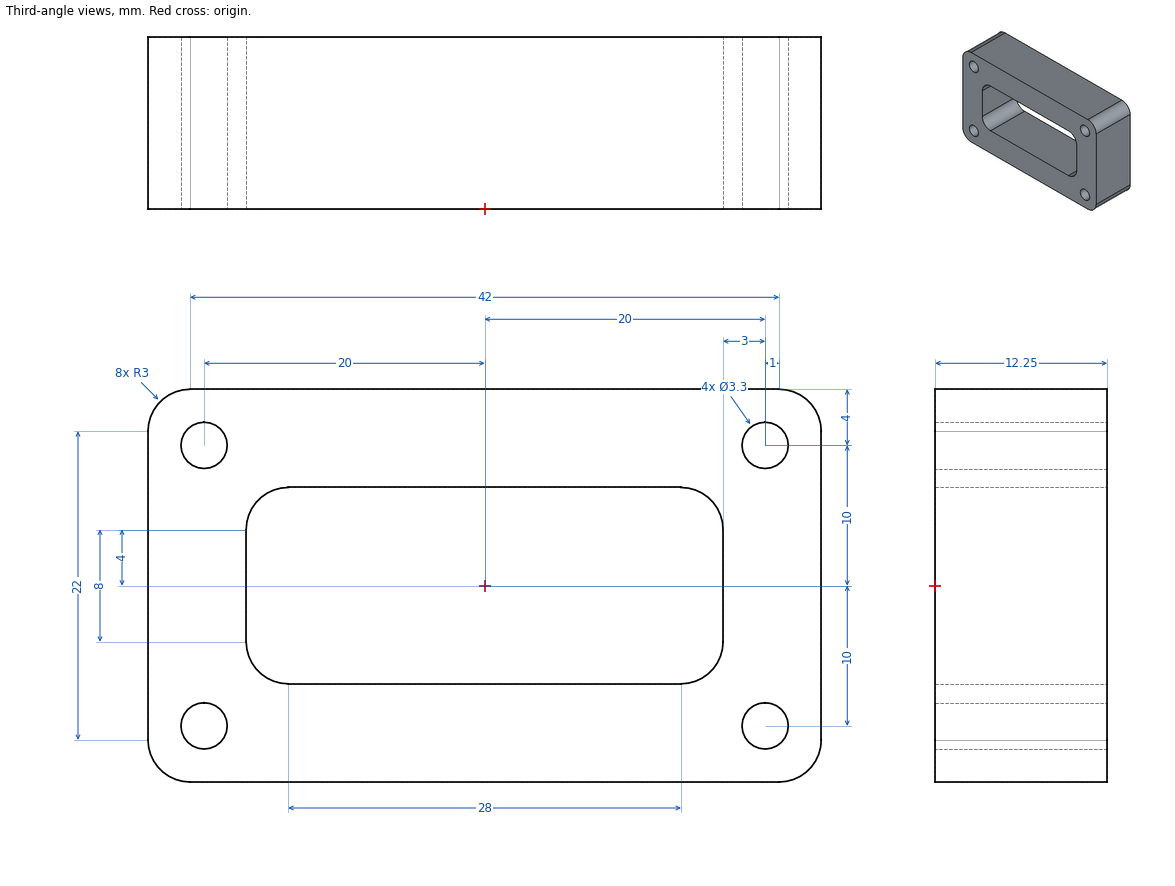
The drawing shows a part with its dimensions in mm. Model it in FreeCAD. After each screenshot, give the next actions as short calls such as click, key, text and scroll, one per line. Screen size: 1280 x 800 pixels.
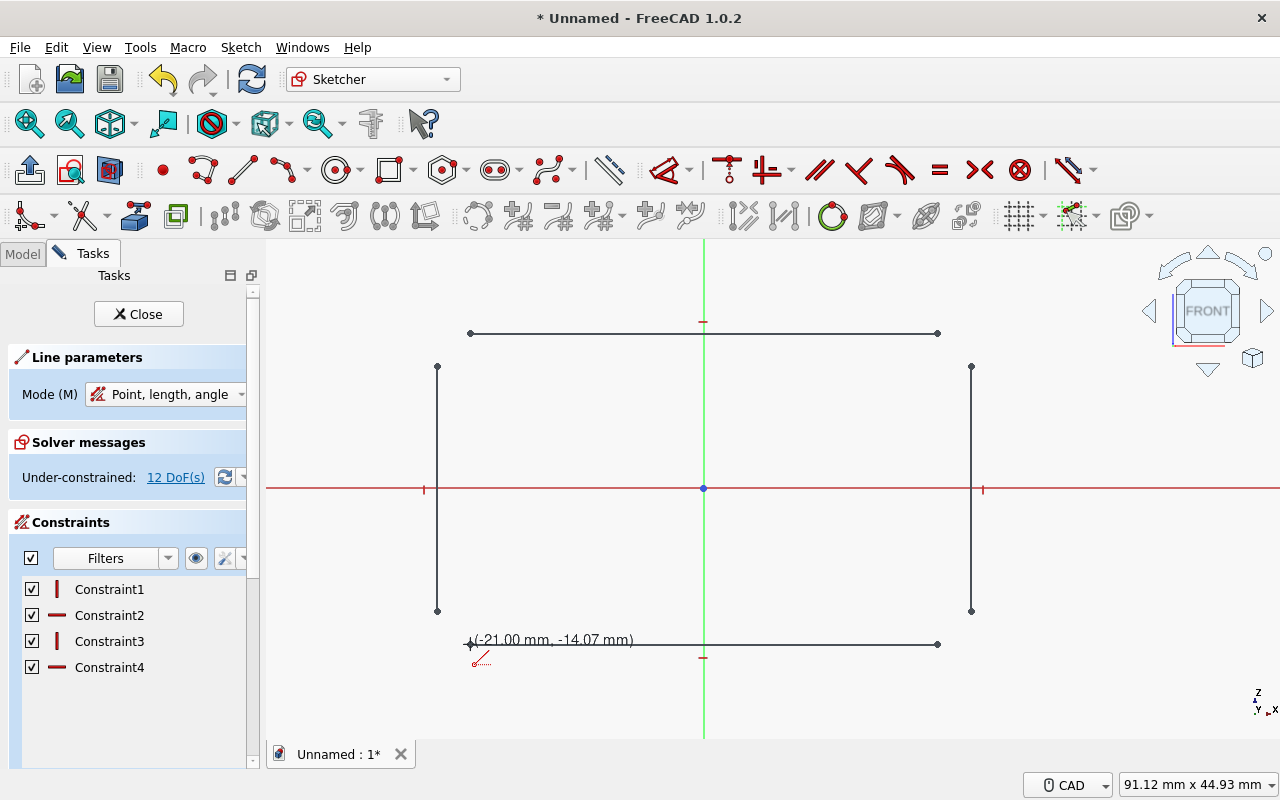
click(284, 170)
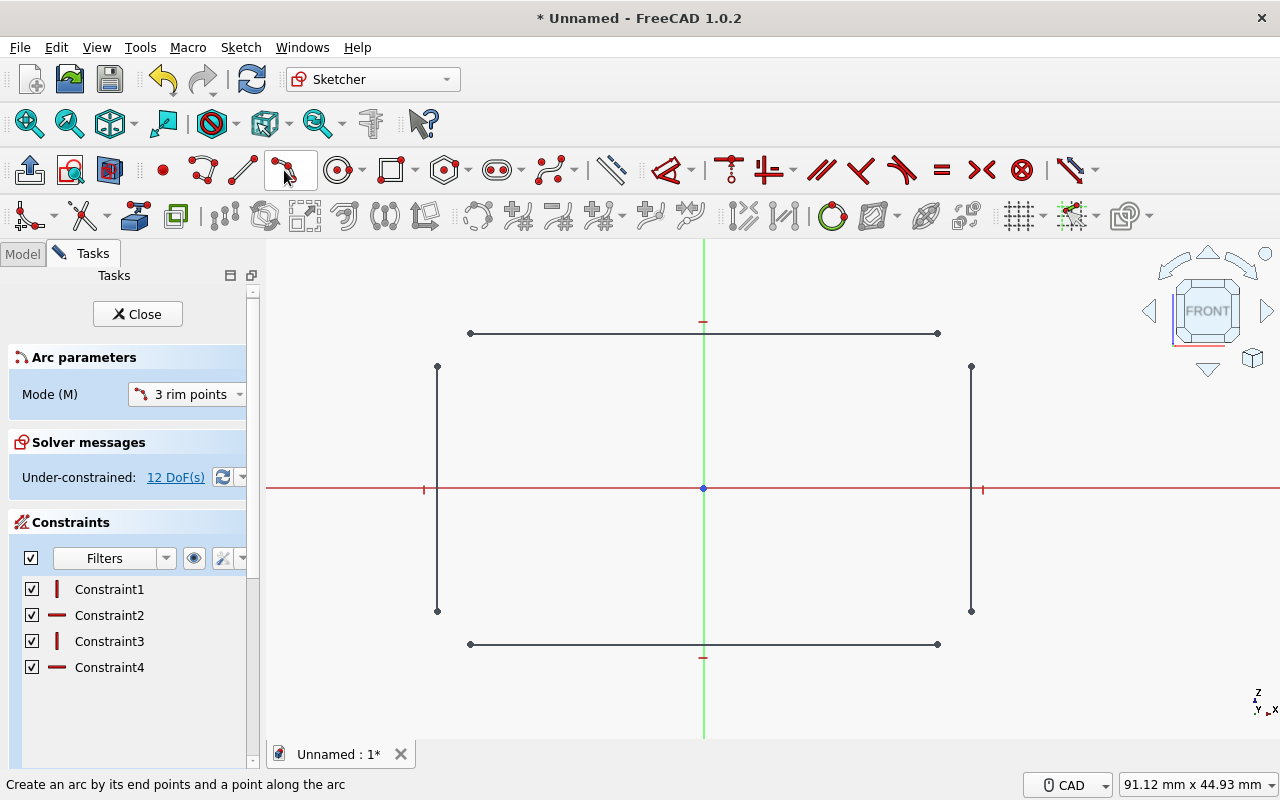
click(437, 367)
click(470, 334)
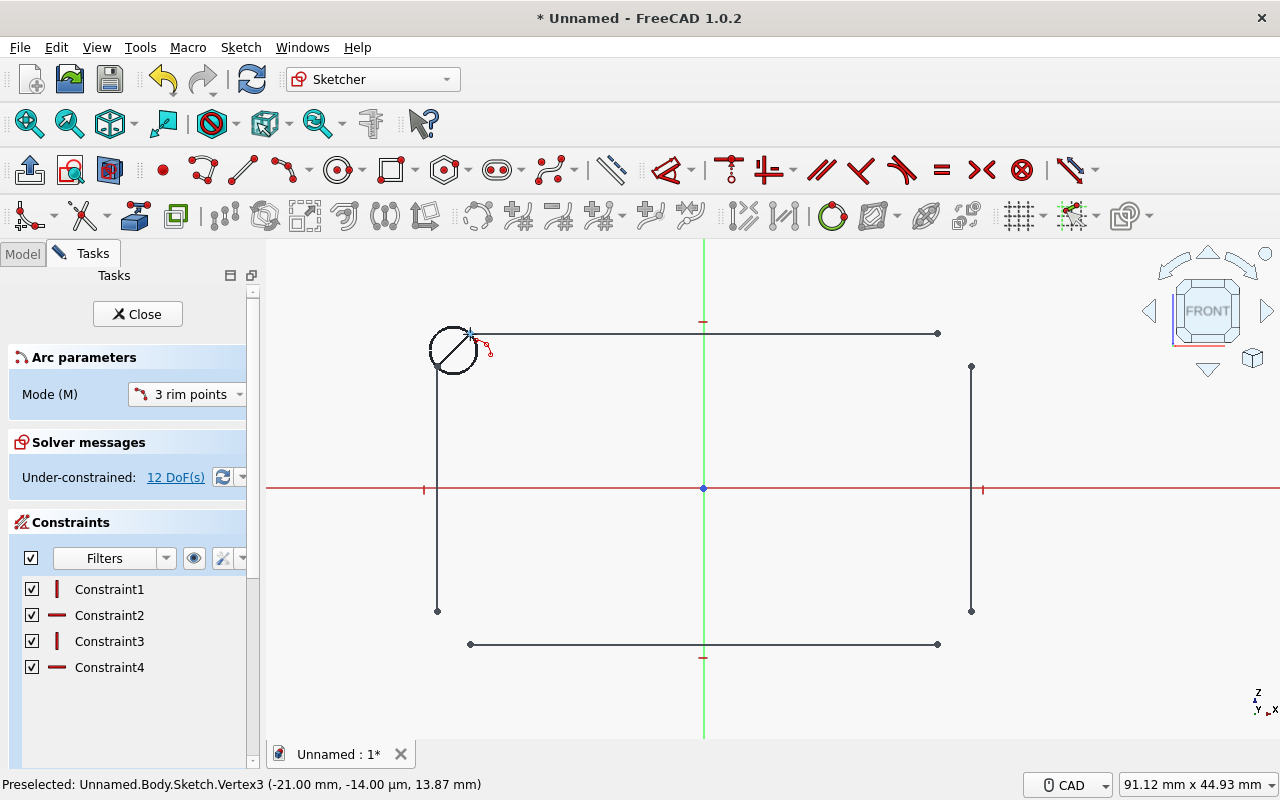
scroll(446, 342, up, 3)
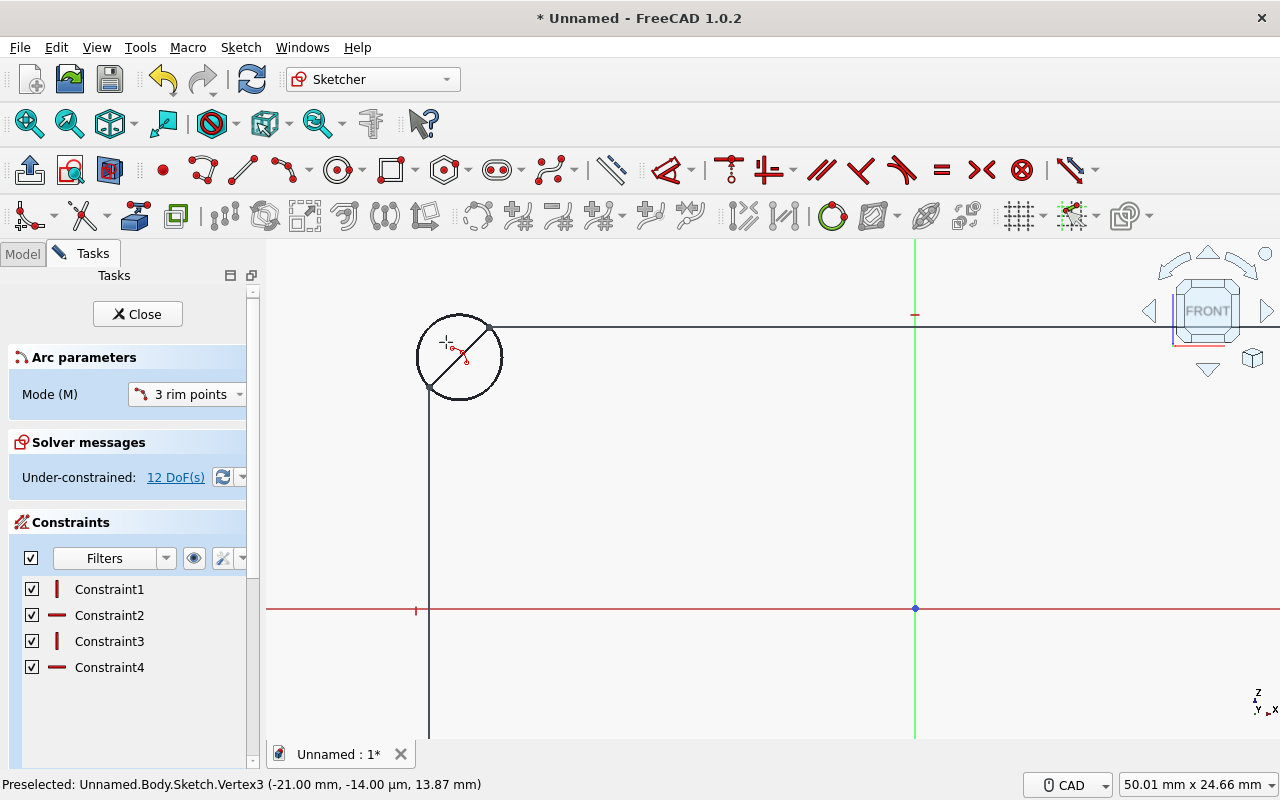
click(447, 343)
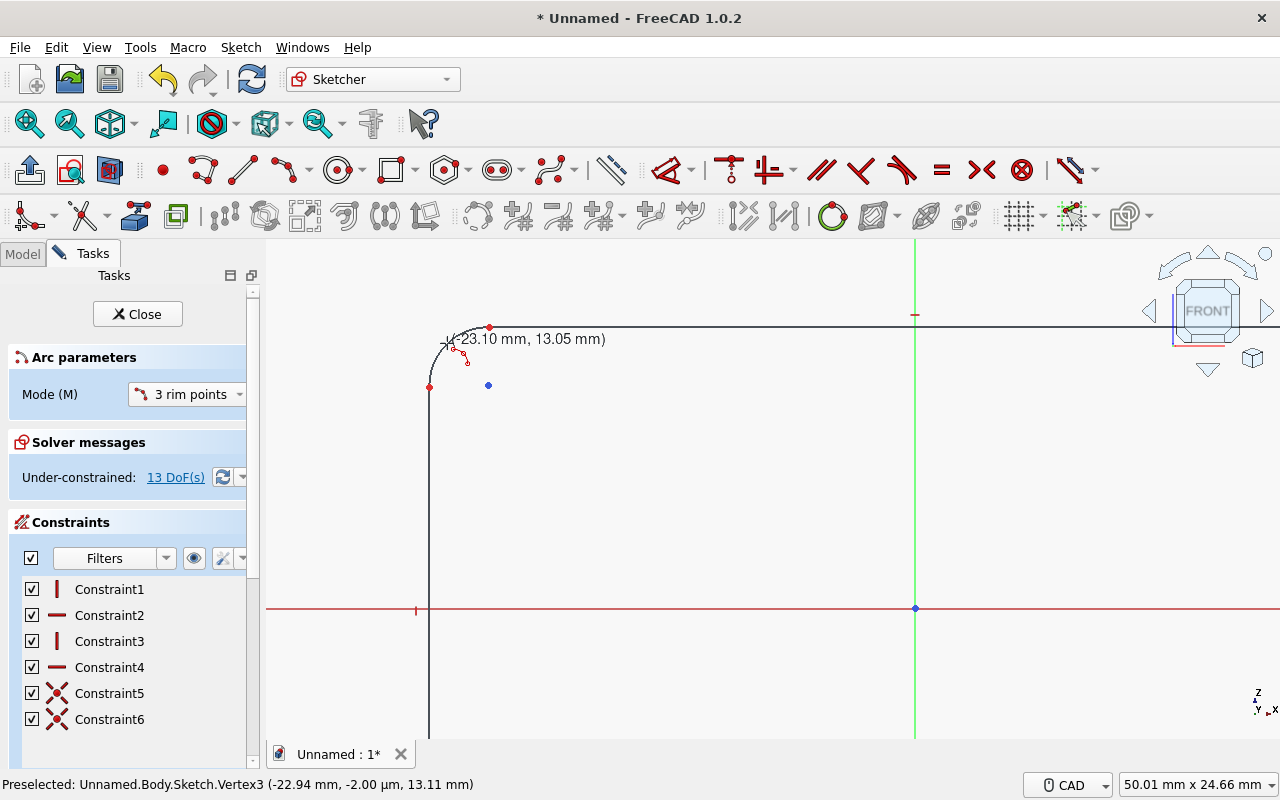
scroll(448, 344, down, 3)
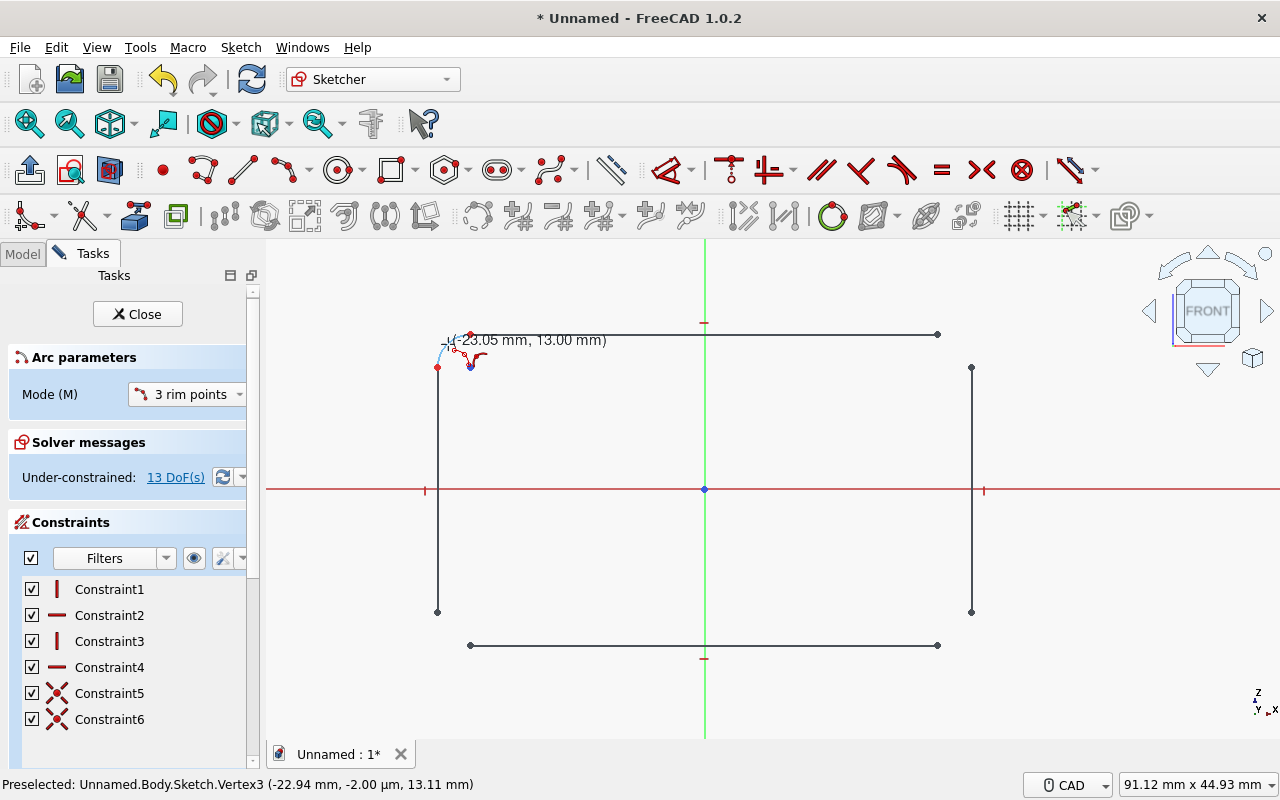
click(938, 335)
click(972, 368)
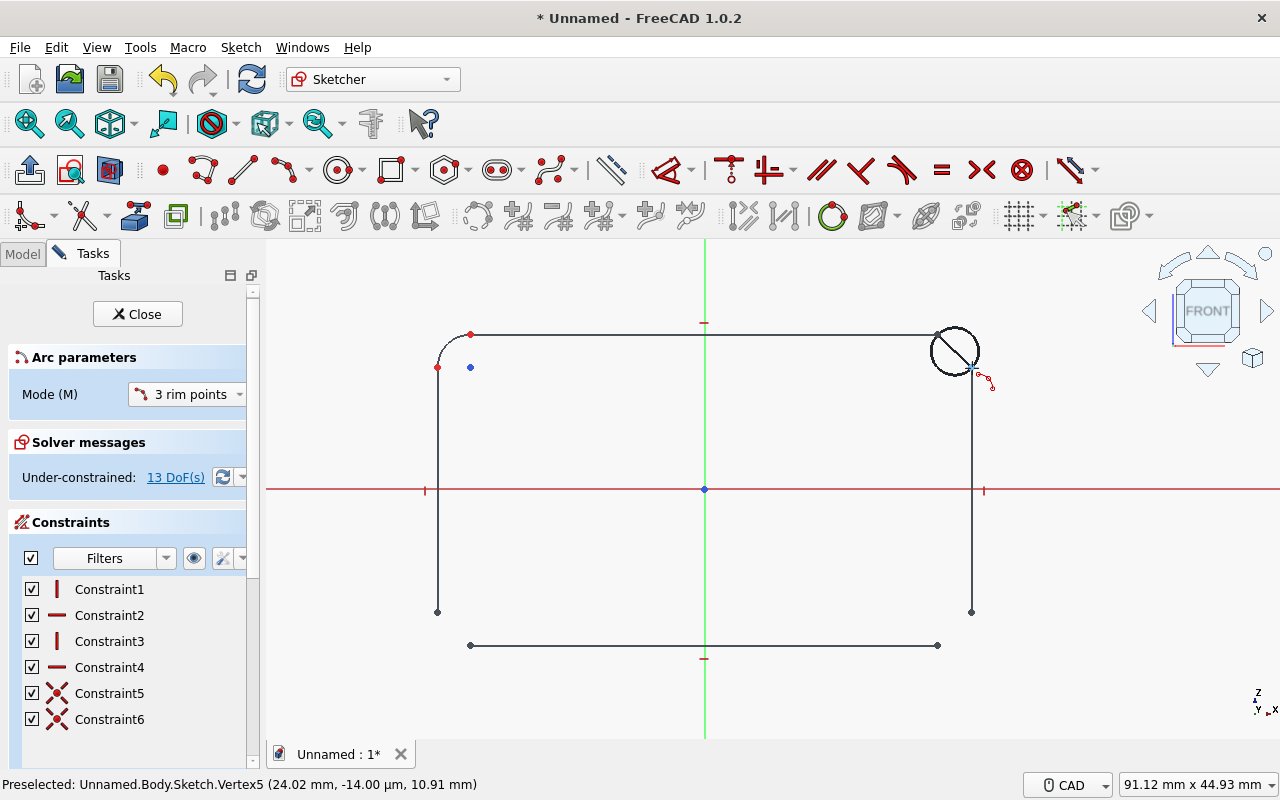
scroll(962, 343, up, 3)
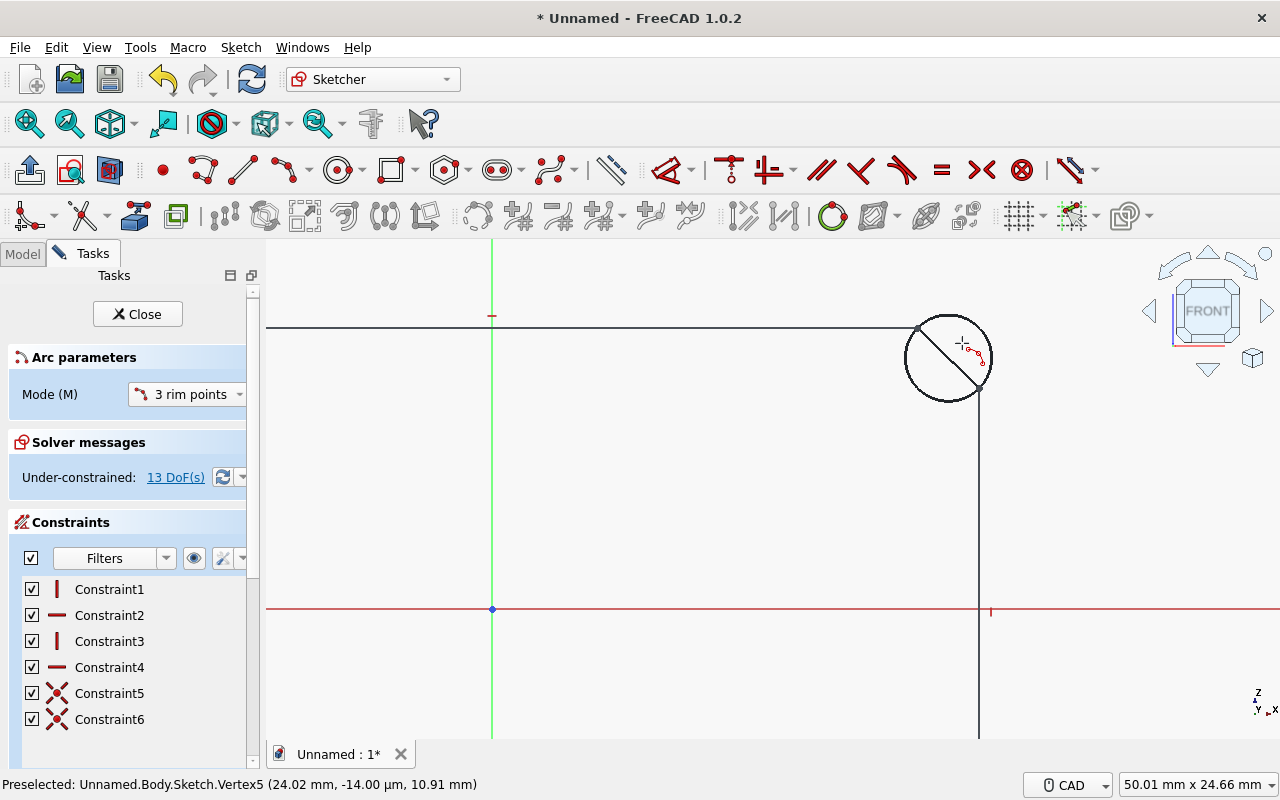
click(961, 343)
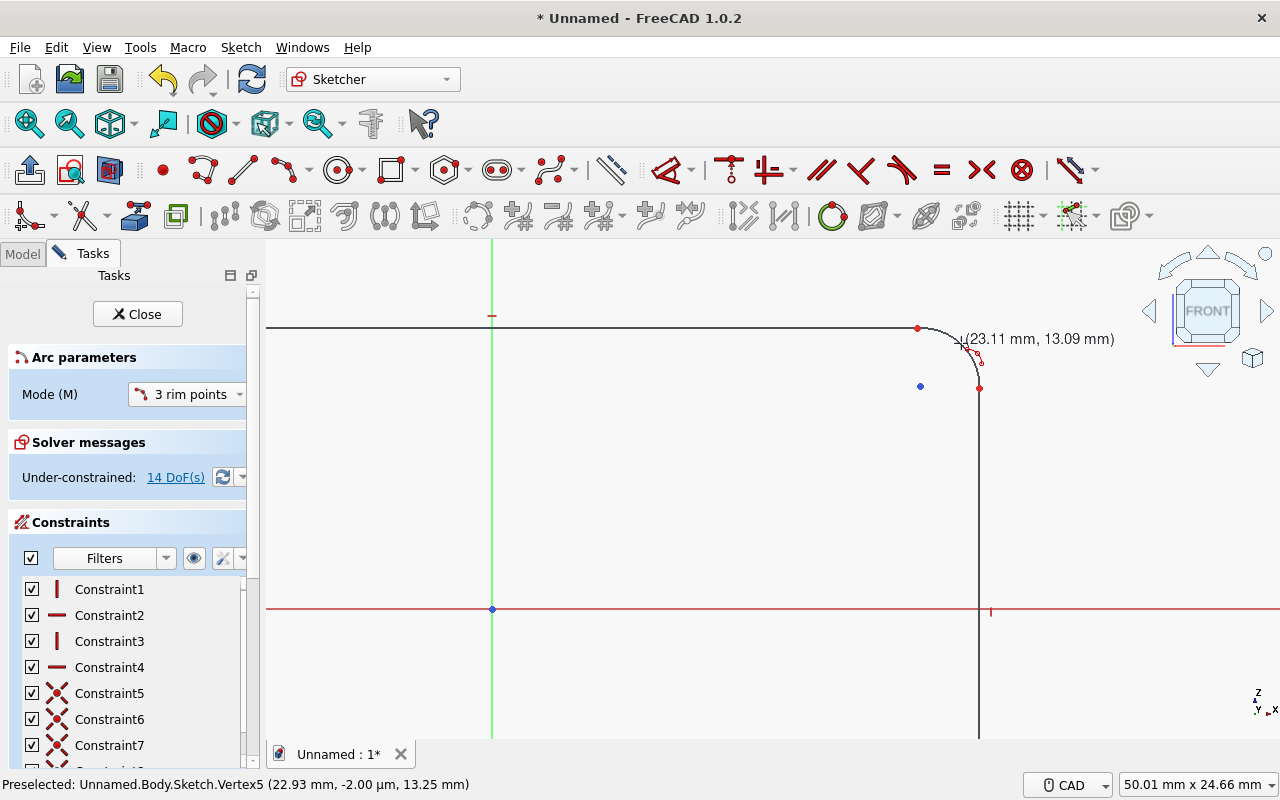
scroll(962, 343, down, 3)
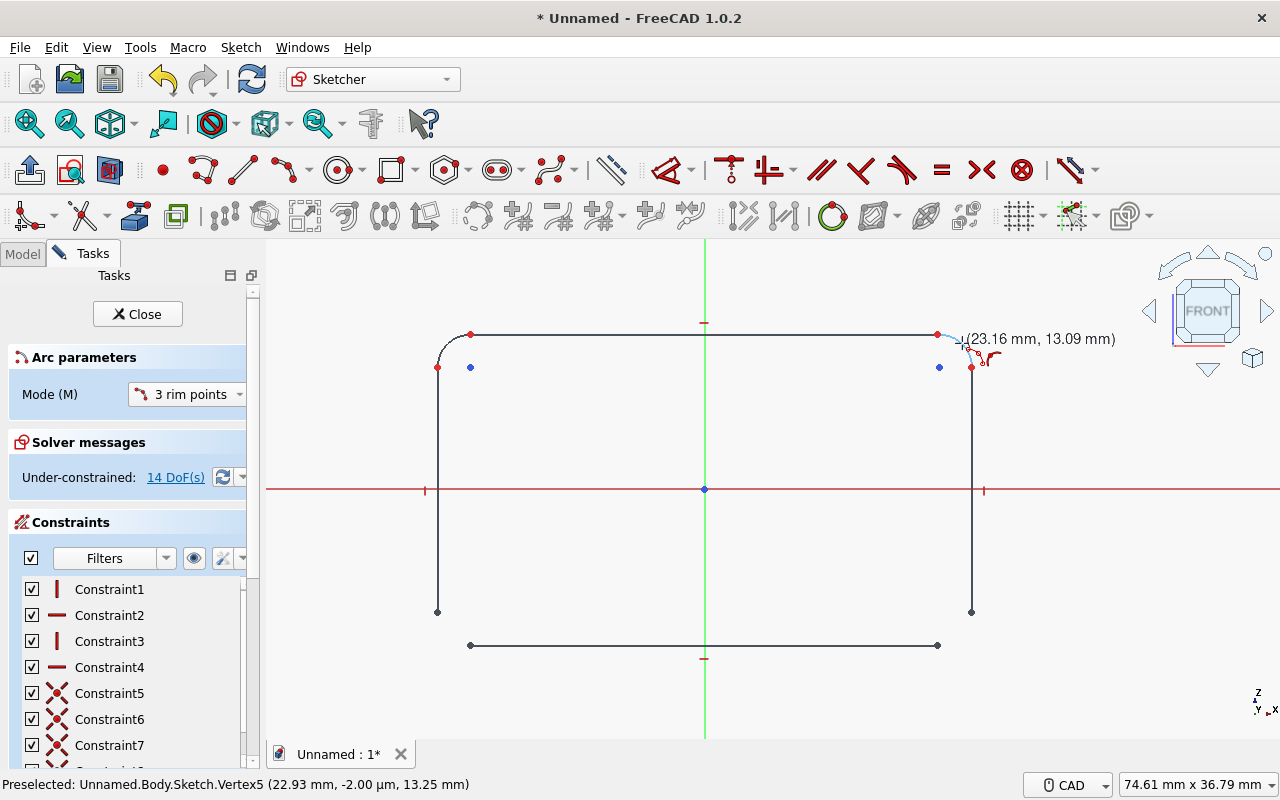
click(972, 613)
click(938, 646)